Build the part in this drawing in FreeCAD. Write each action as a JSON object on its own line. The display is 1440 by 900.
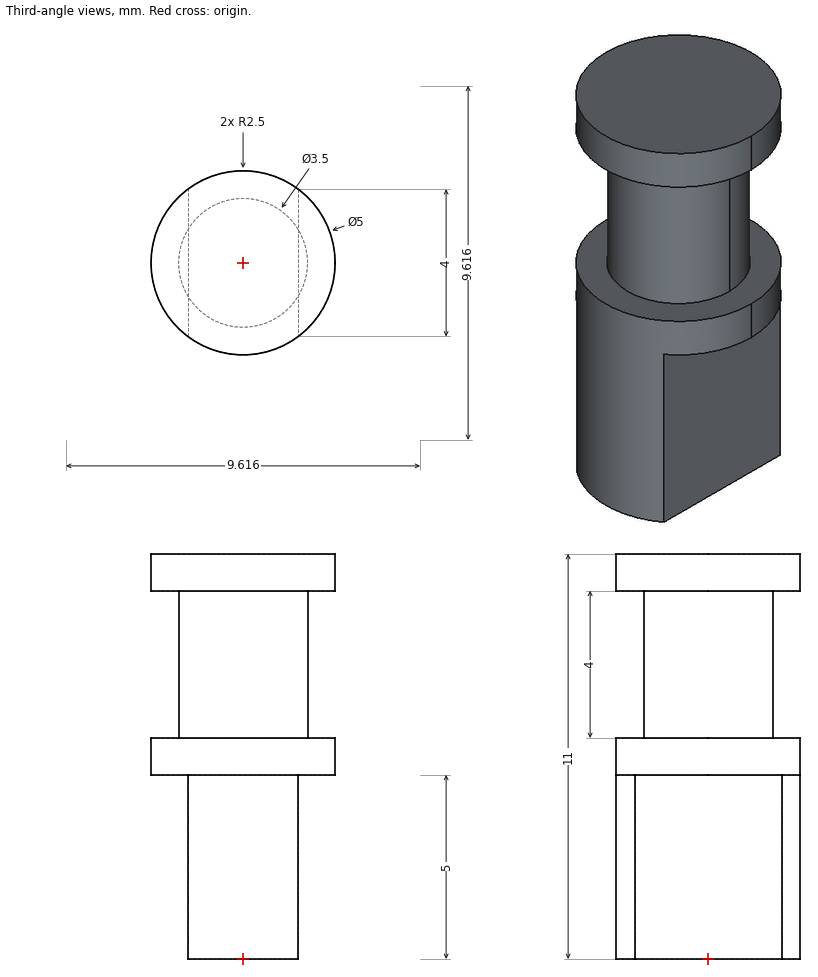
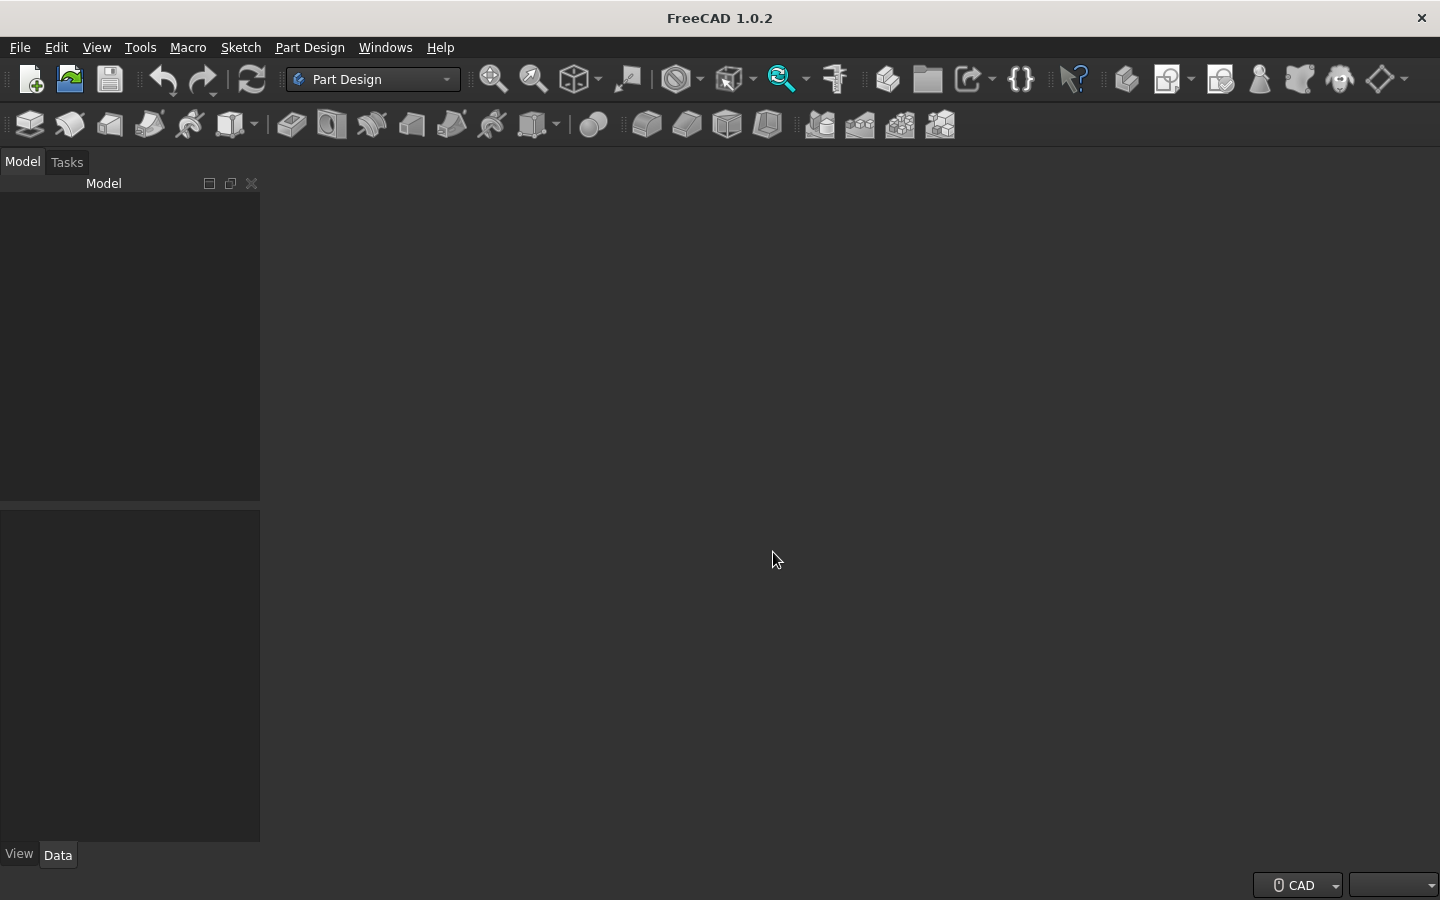
{"action": "key", "text": "ctrl+n"}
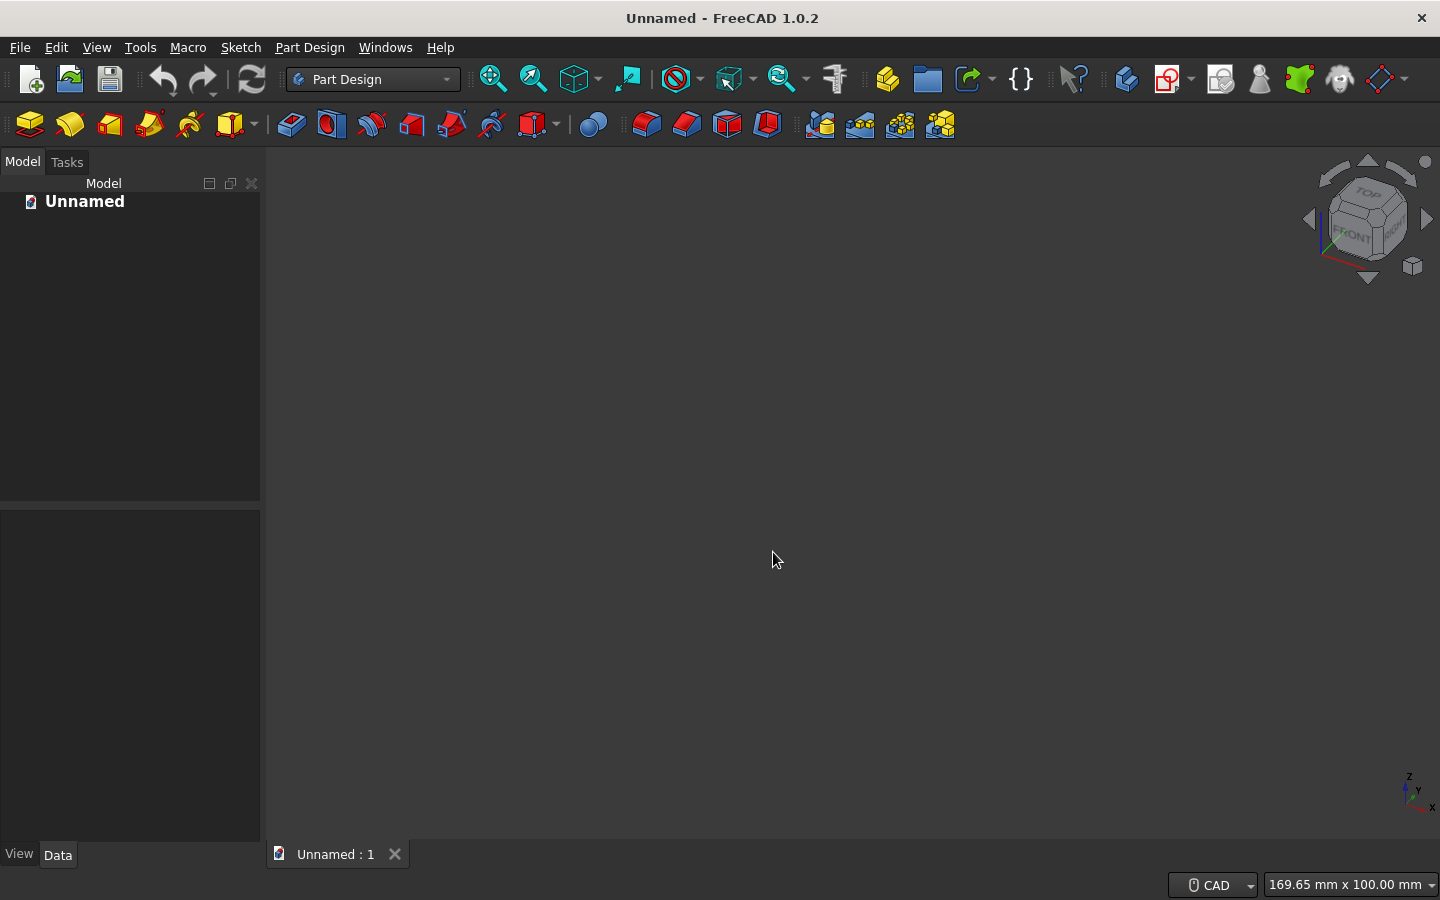
{"action": "left_click", "coordinate": [1168, 80]}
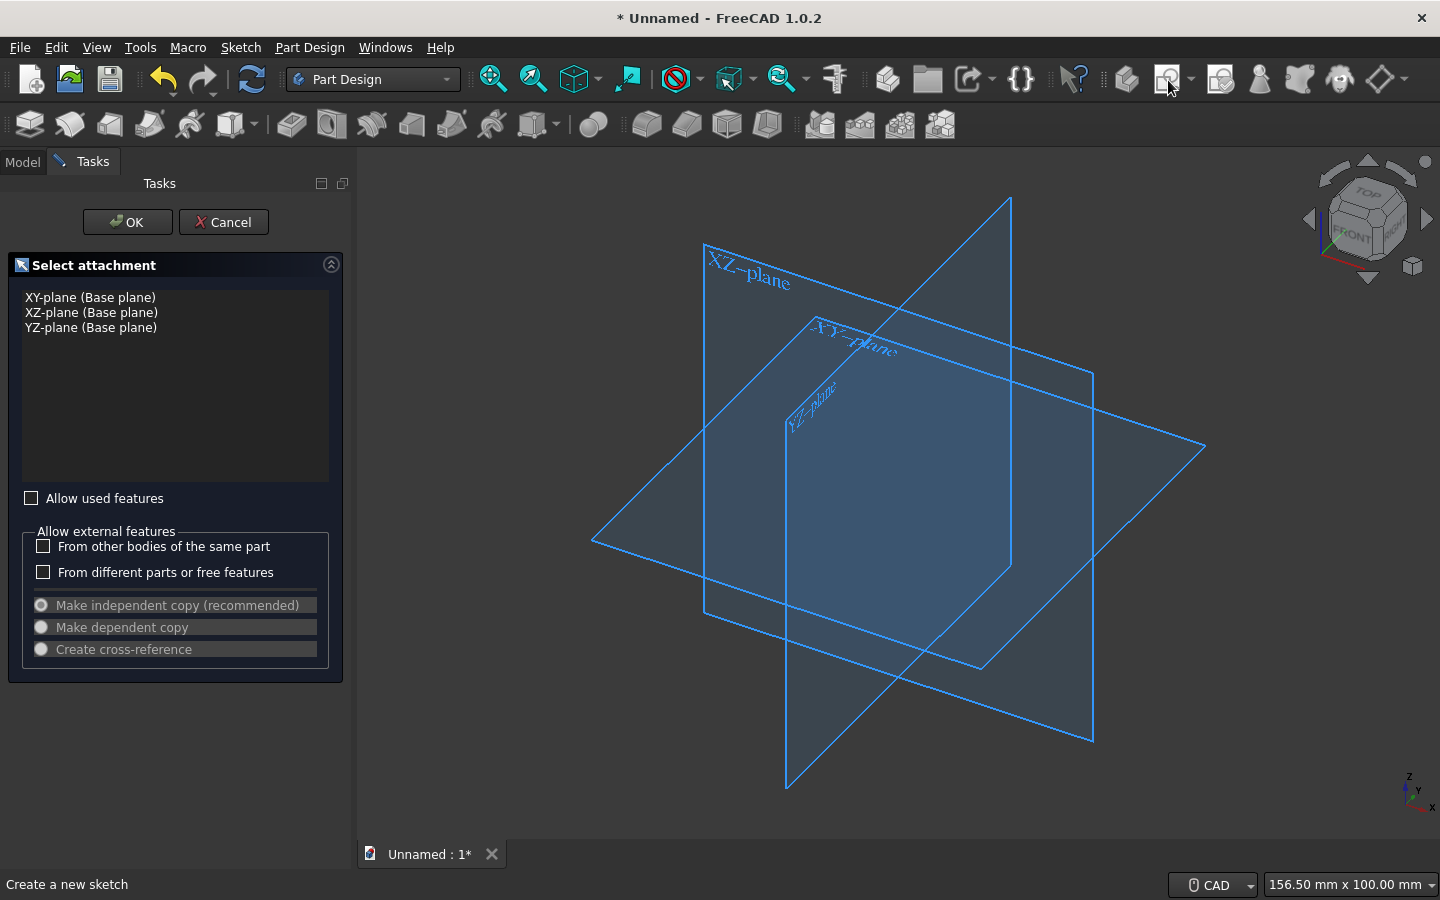
{"action": "left_click", "coordinate": [82, 298]}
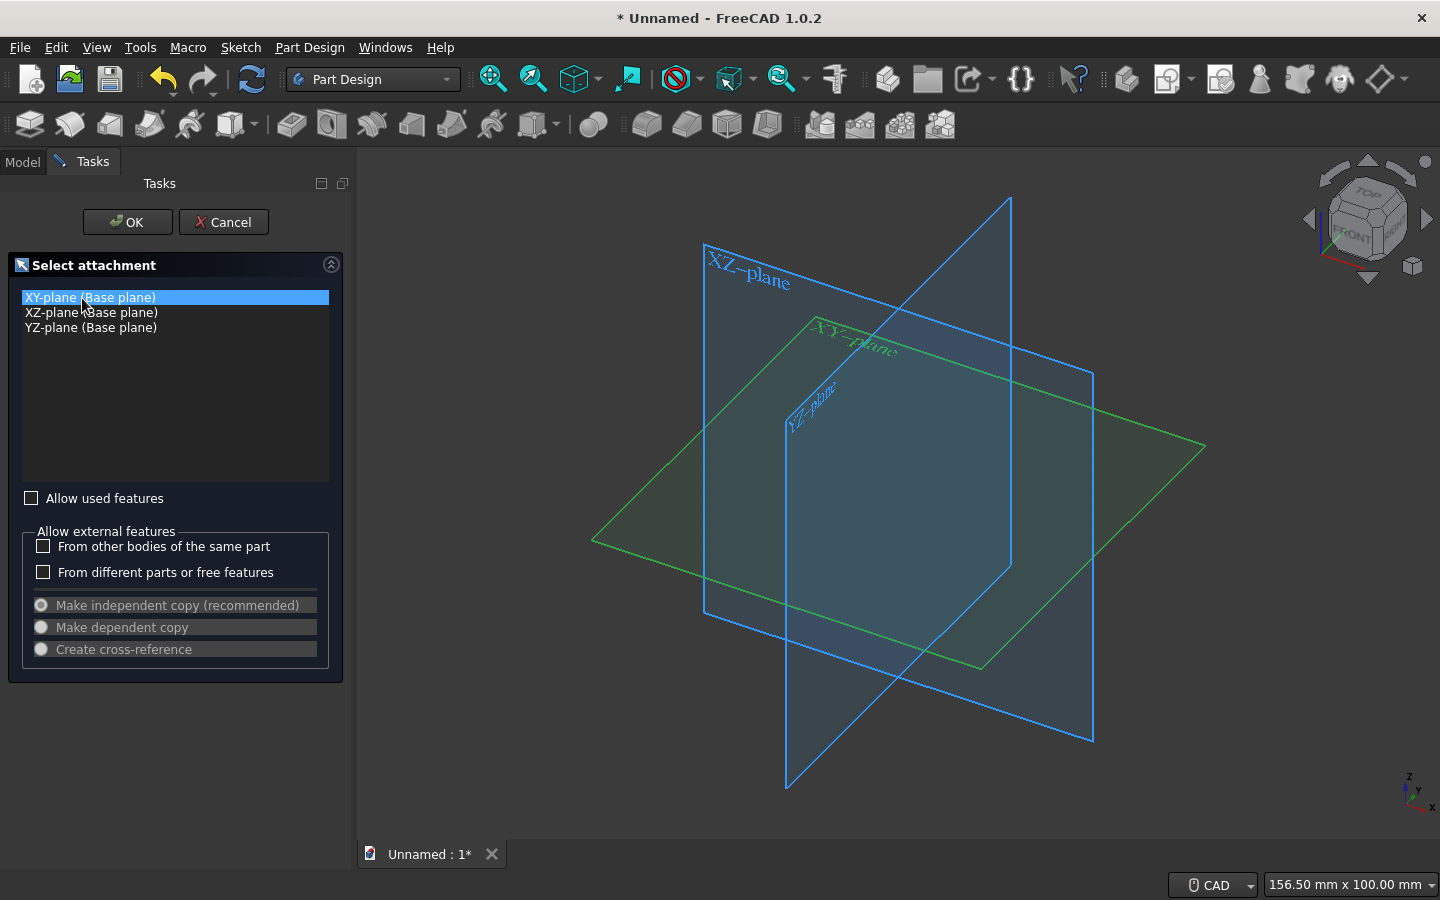
{"action": "left_click", "coordinate": [128, 222]}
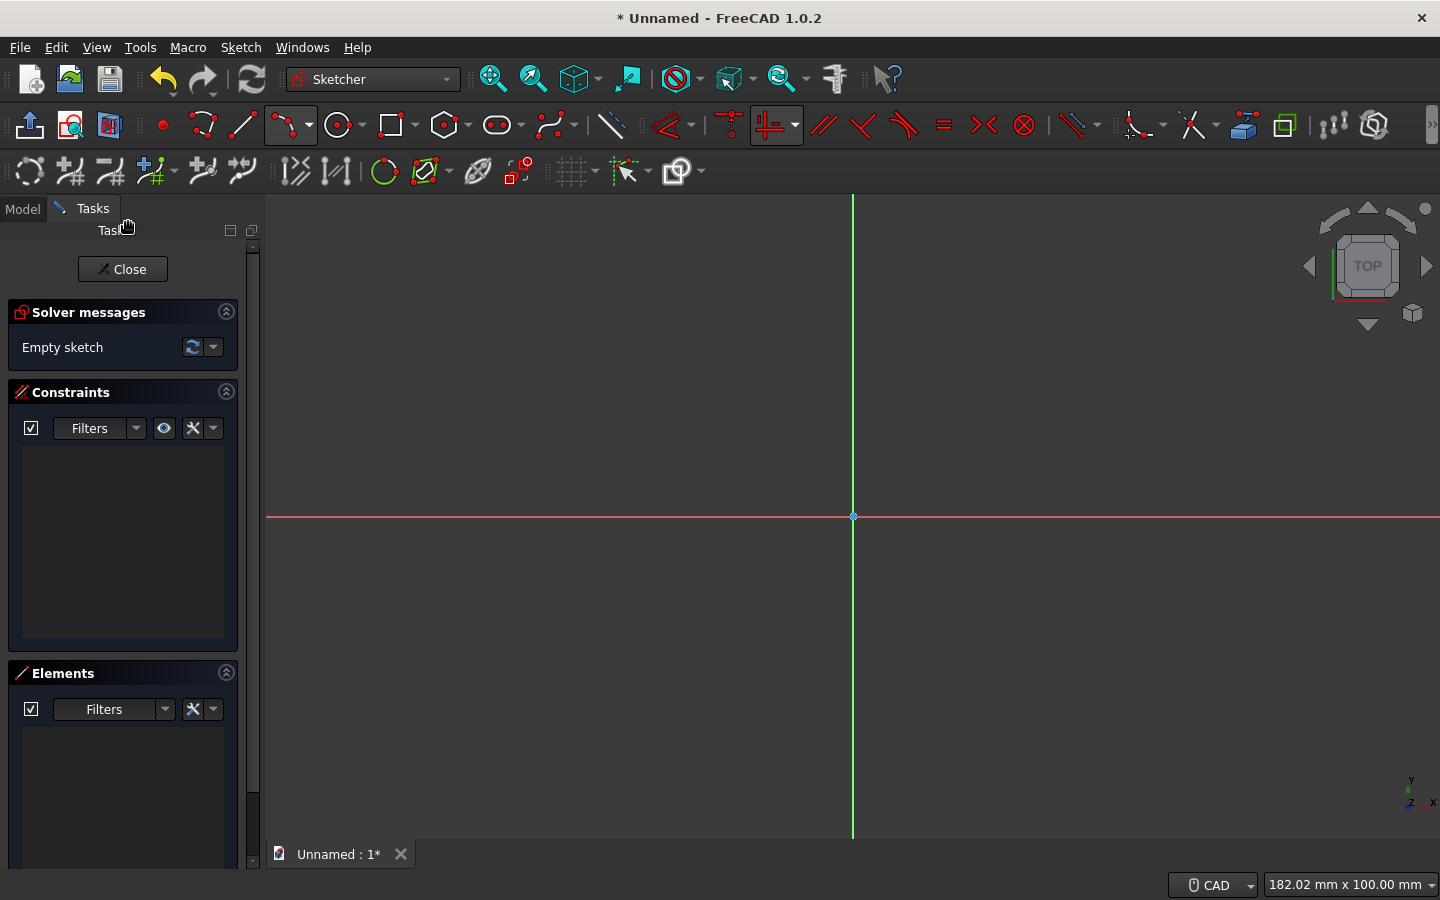
{"action": "scroll", "coordinate": [858, 516], "scroll_direction": "up", "scroll_amount": 13}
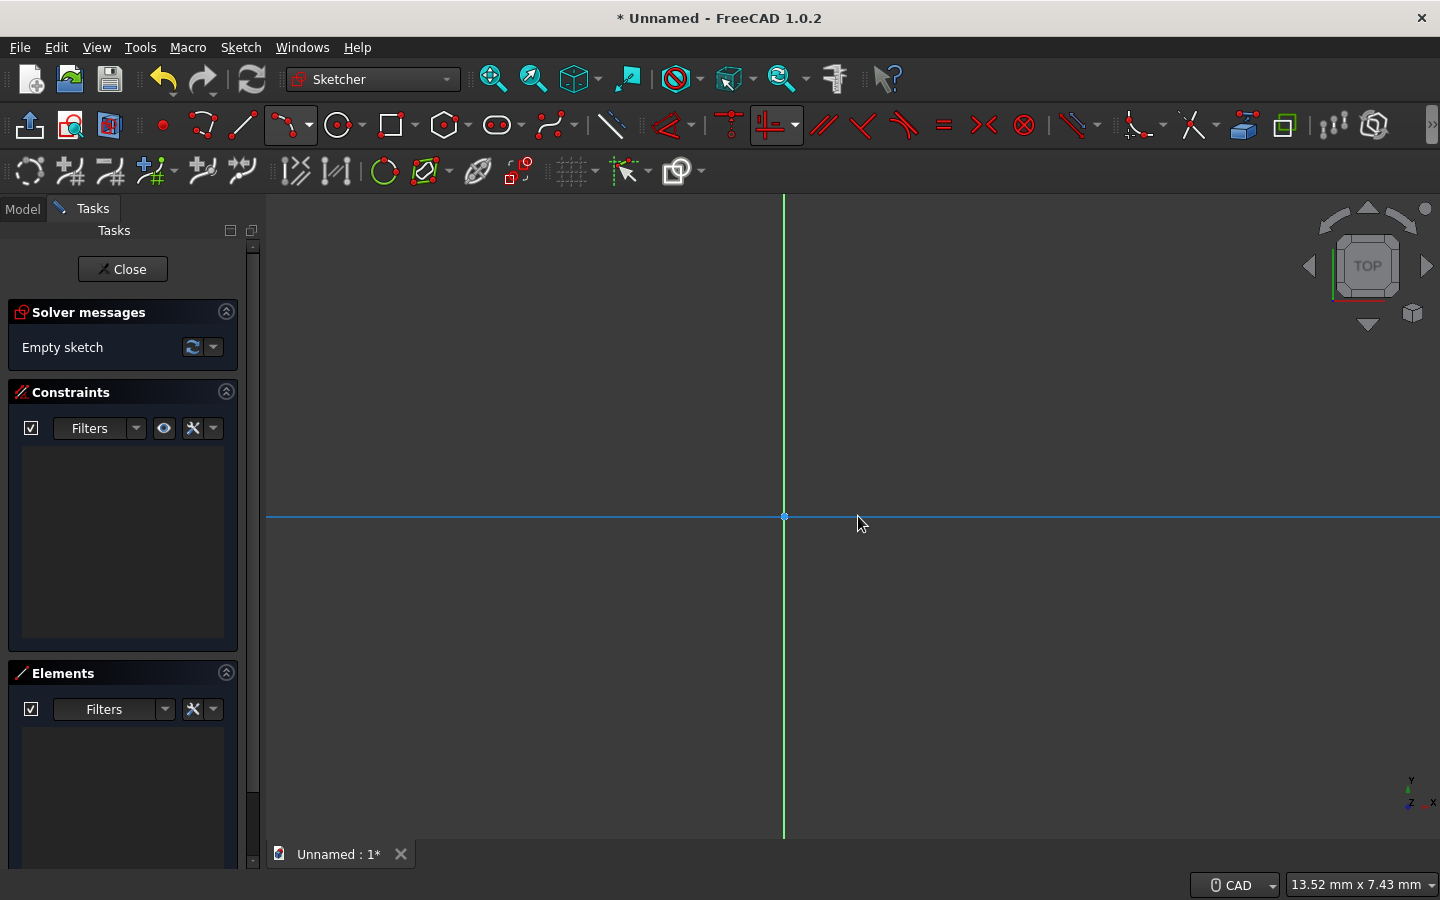
{"action": "key", "text": "g c"}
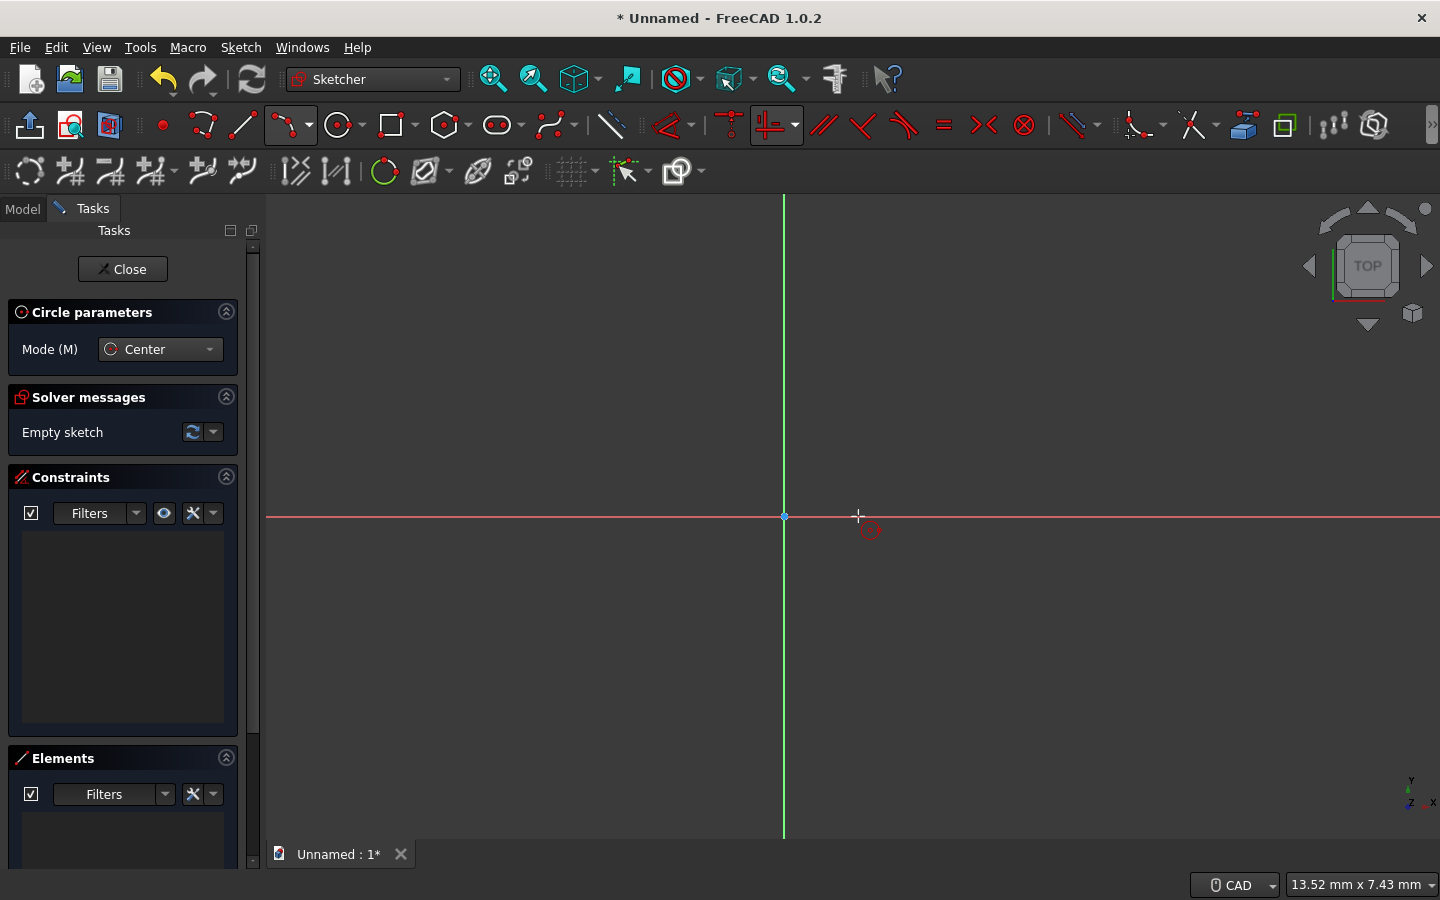
{"action": "left_click", "coordinate": [784, 516]}
{"action": "mouse_move", "coordinate": [938, 363]}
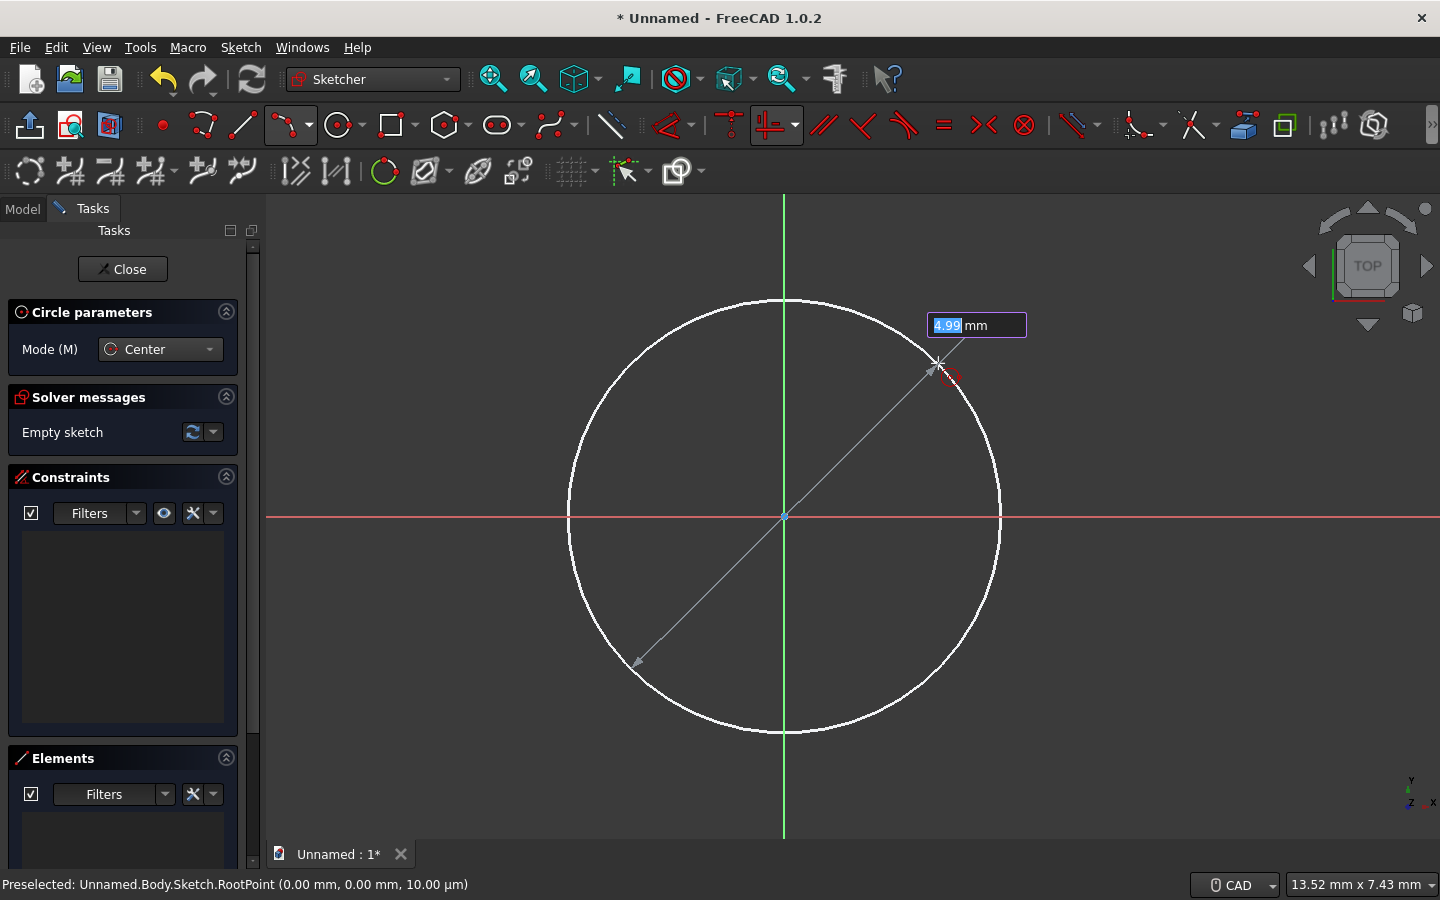
{"action": "type", "text": "5"}
{"action": "key", "text": "Return"}
{"action": "key", "text": "Escape"}